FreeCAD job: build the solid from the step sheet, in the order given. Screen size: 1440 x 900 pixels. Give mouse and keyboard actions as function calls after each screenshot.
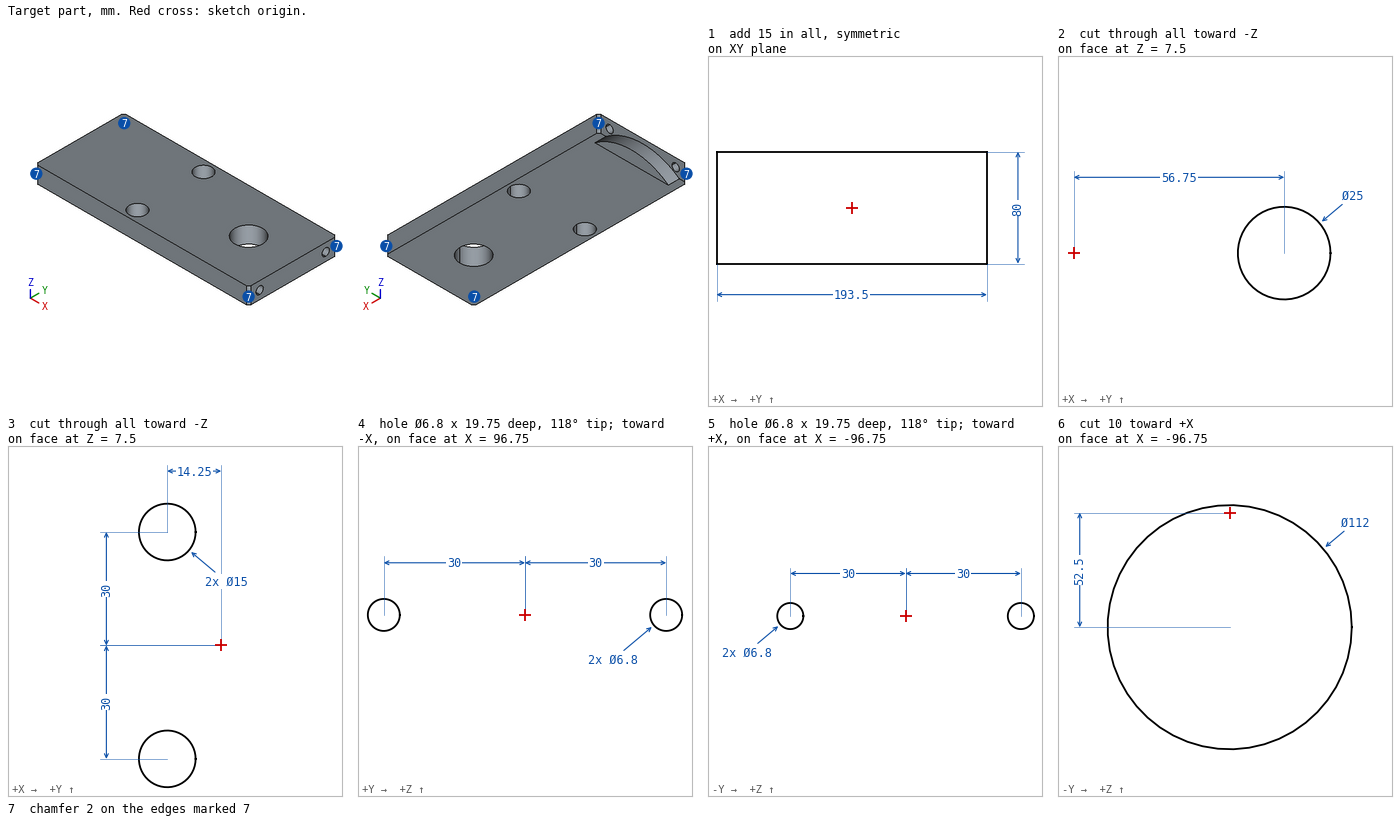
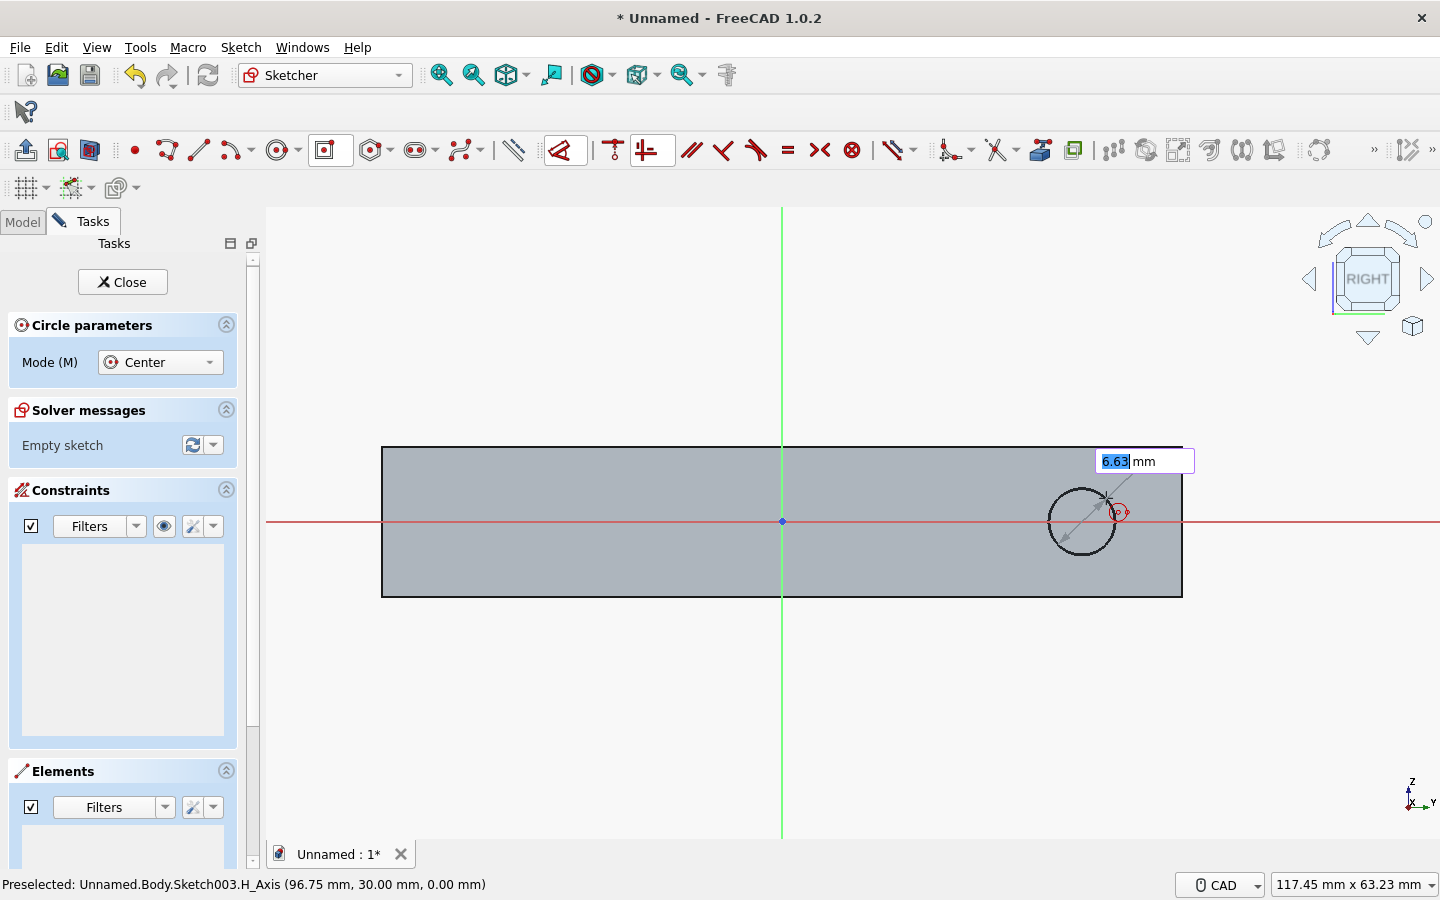
text(6.8)
key(Return)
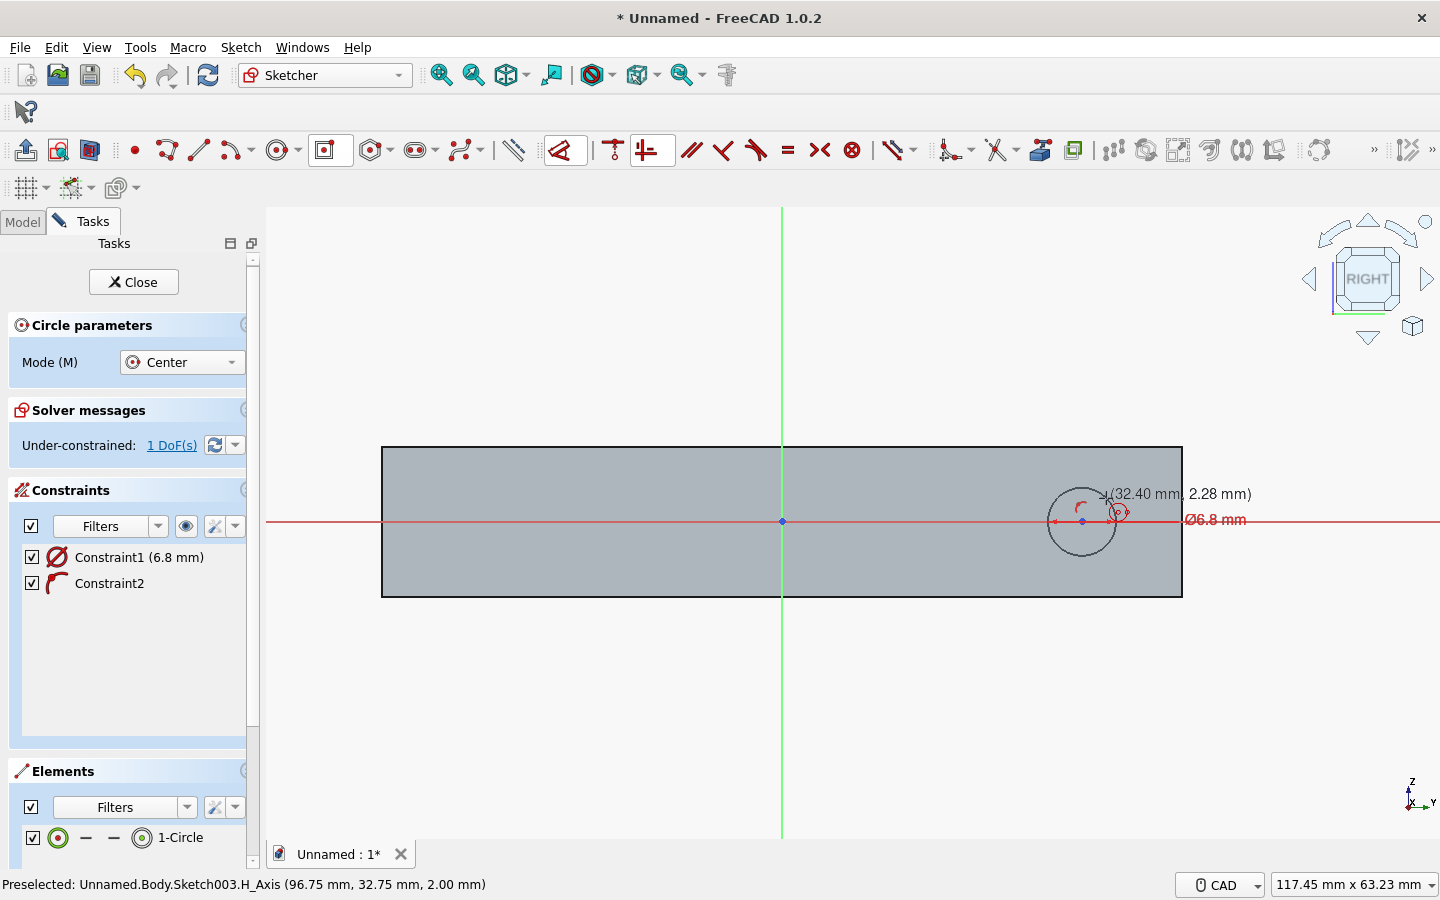
click(482, 522)
move(506, 498)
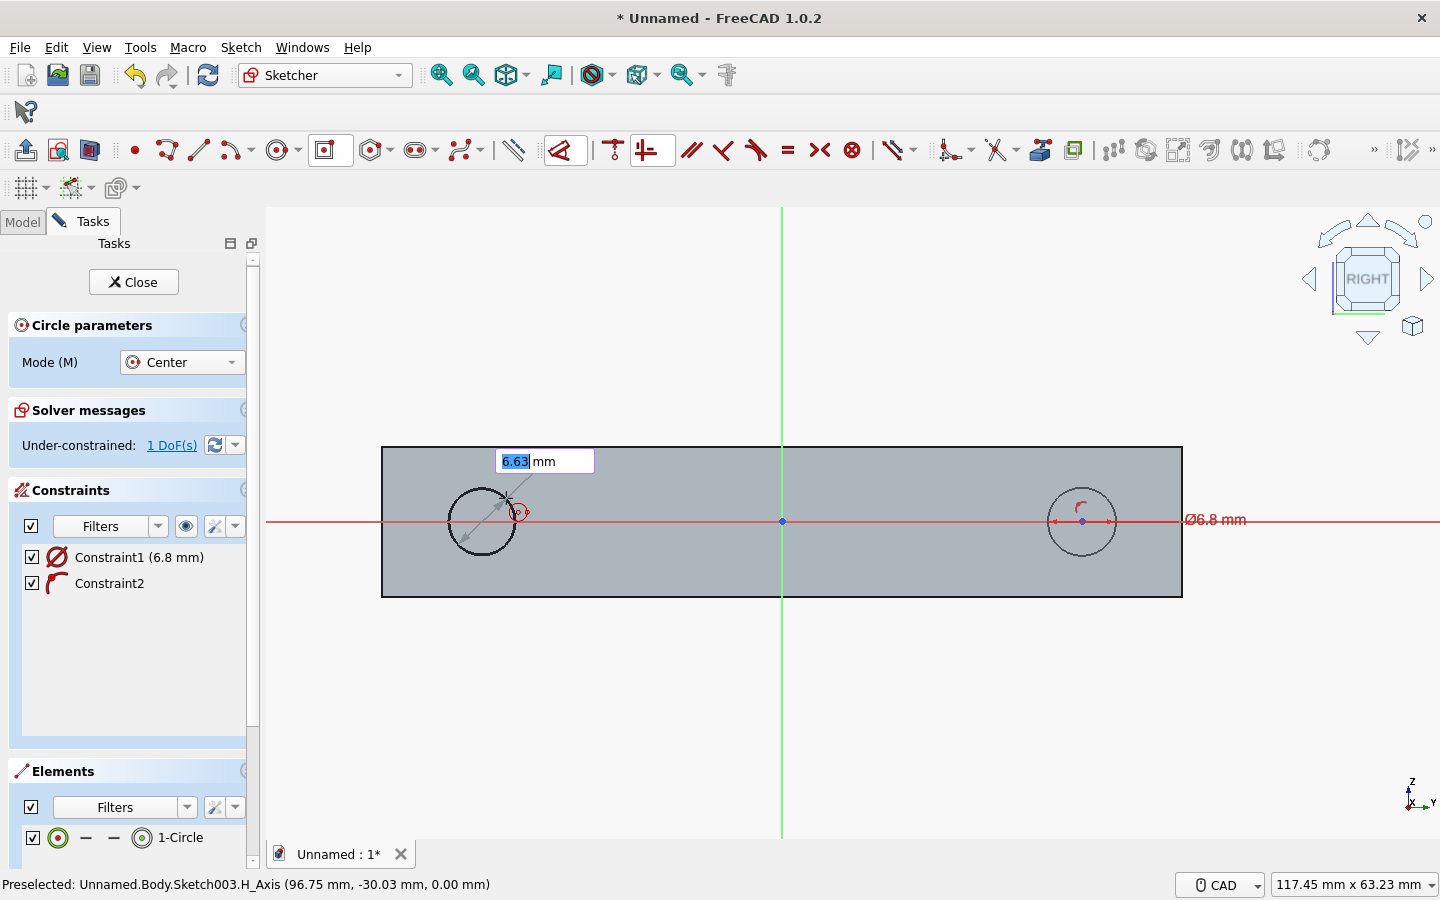
text(6.8)
key(Return)
key(Escape)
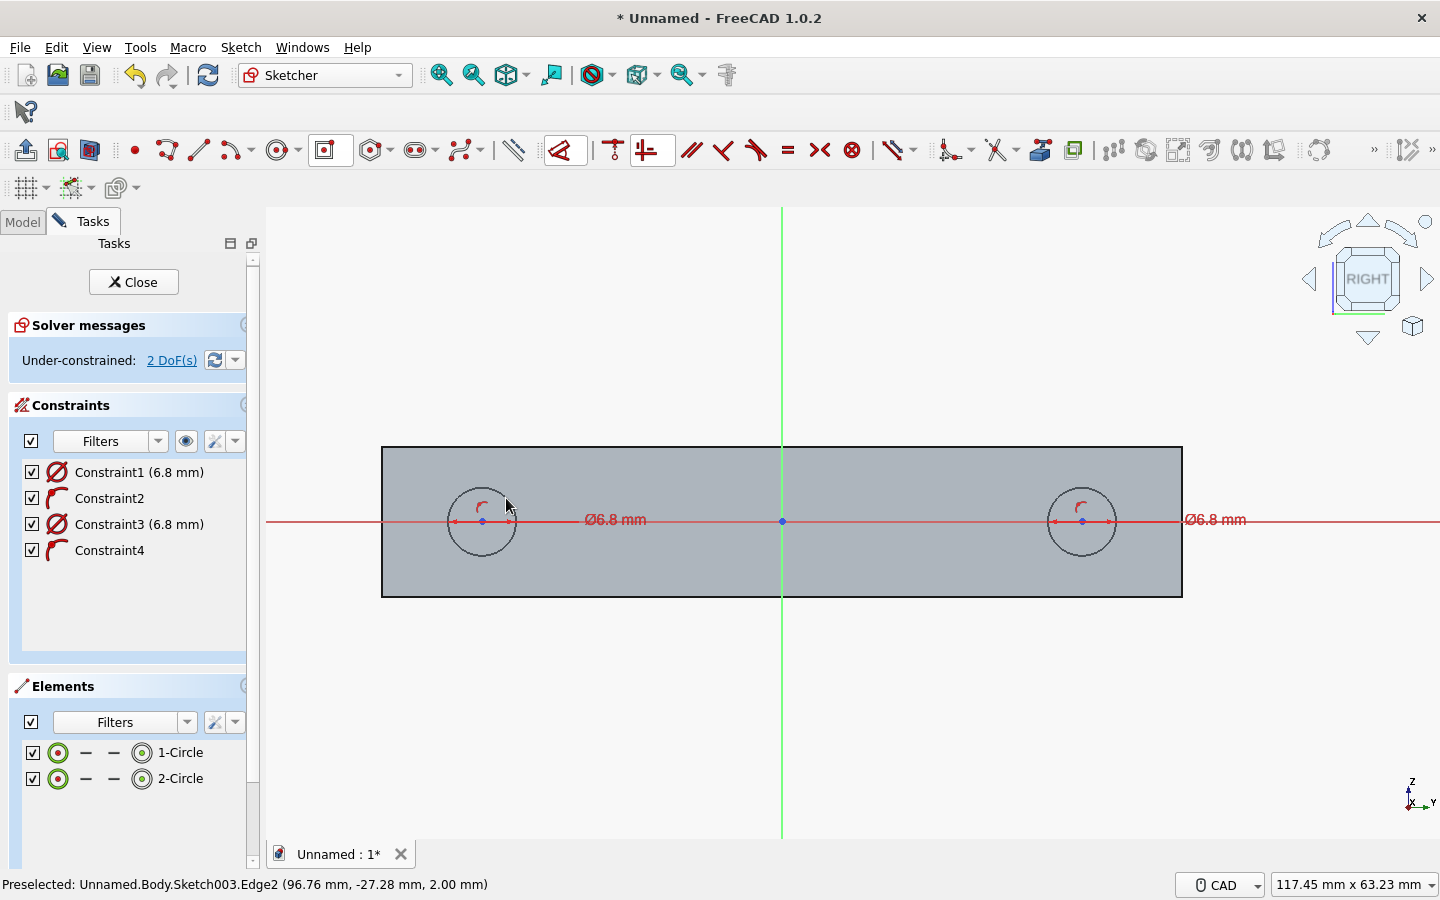
click(1082, 522)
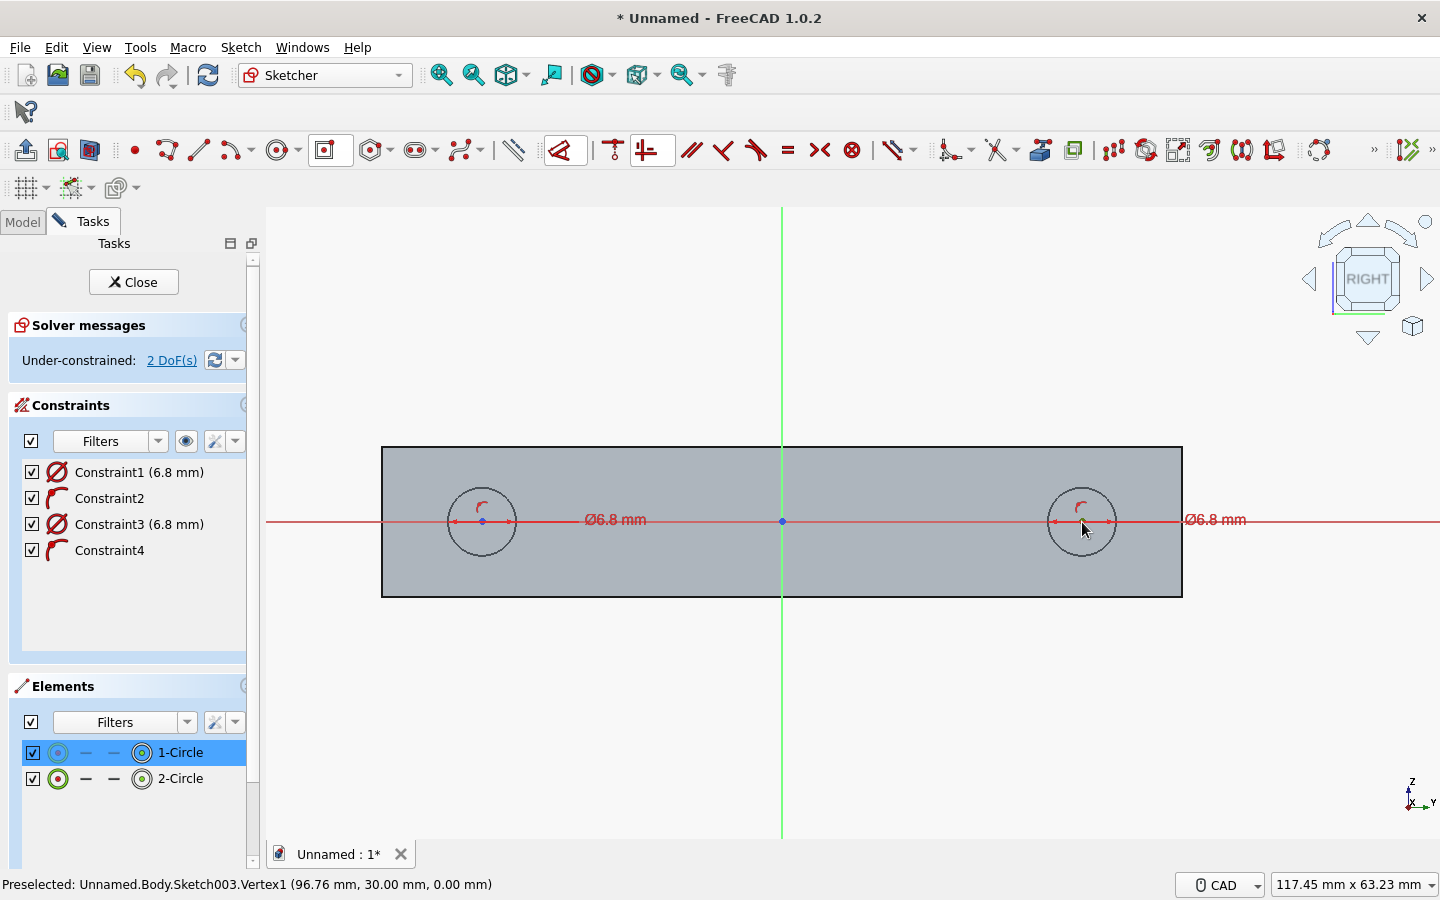
key(l)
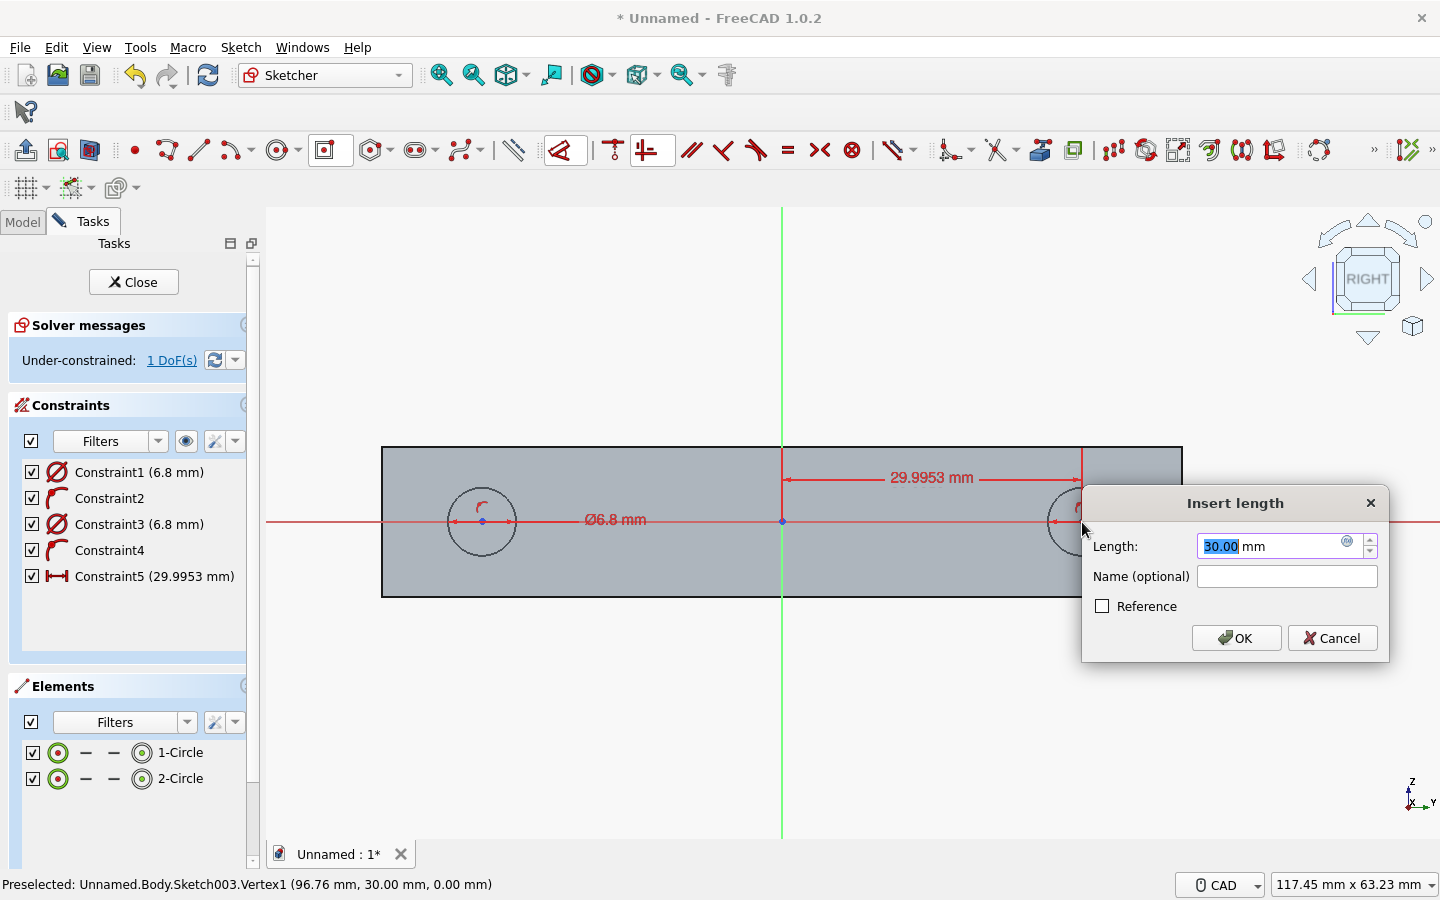
text(30)
key(Return)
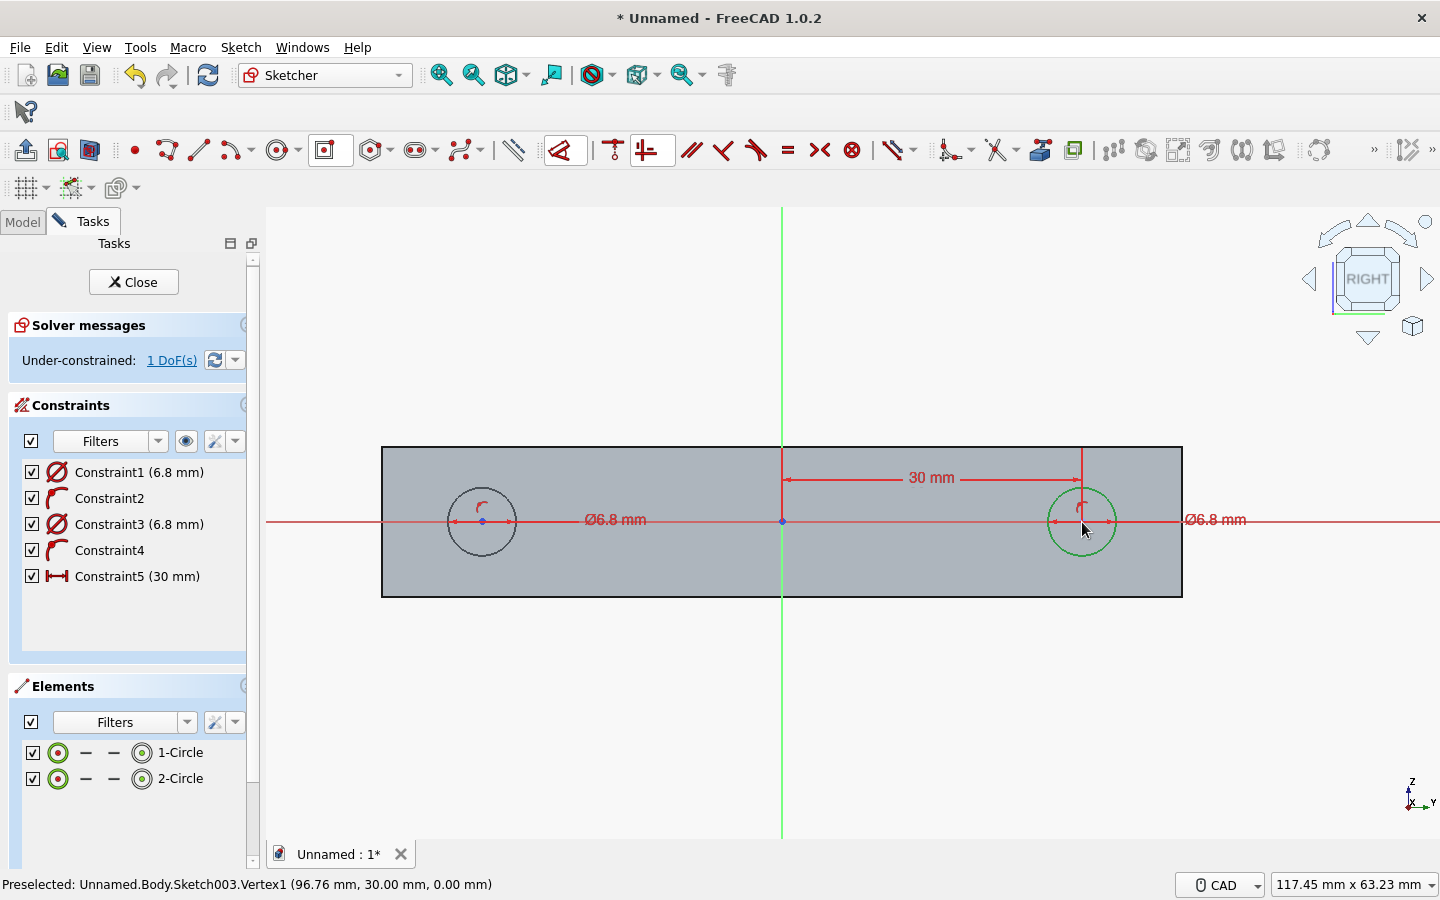
click(482, 522)